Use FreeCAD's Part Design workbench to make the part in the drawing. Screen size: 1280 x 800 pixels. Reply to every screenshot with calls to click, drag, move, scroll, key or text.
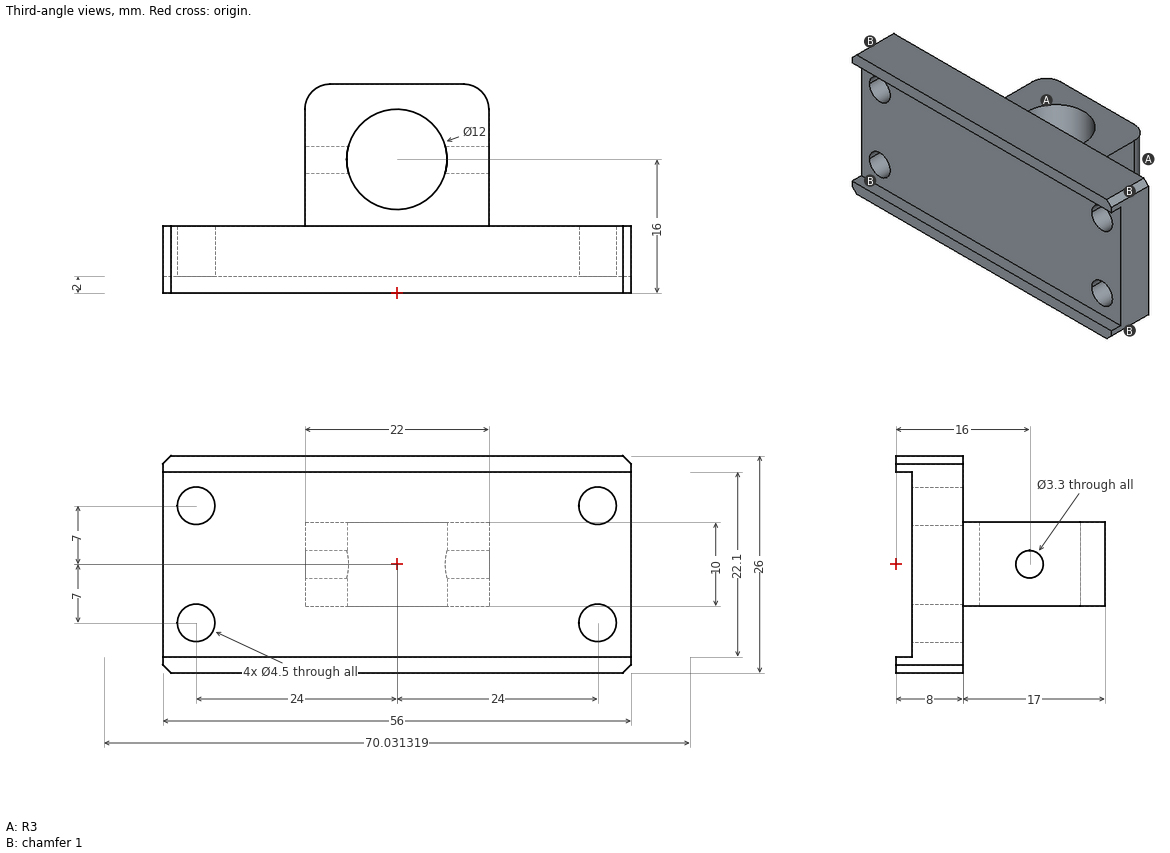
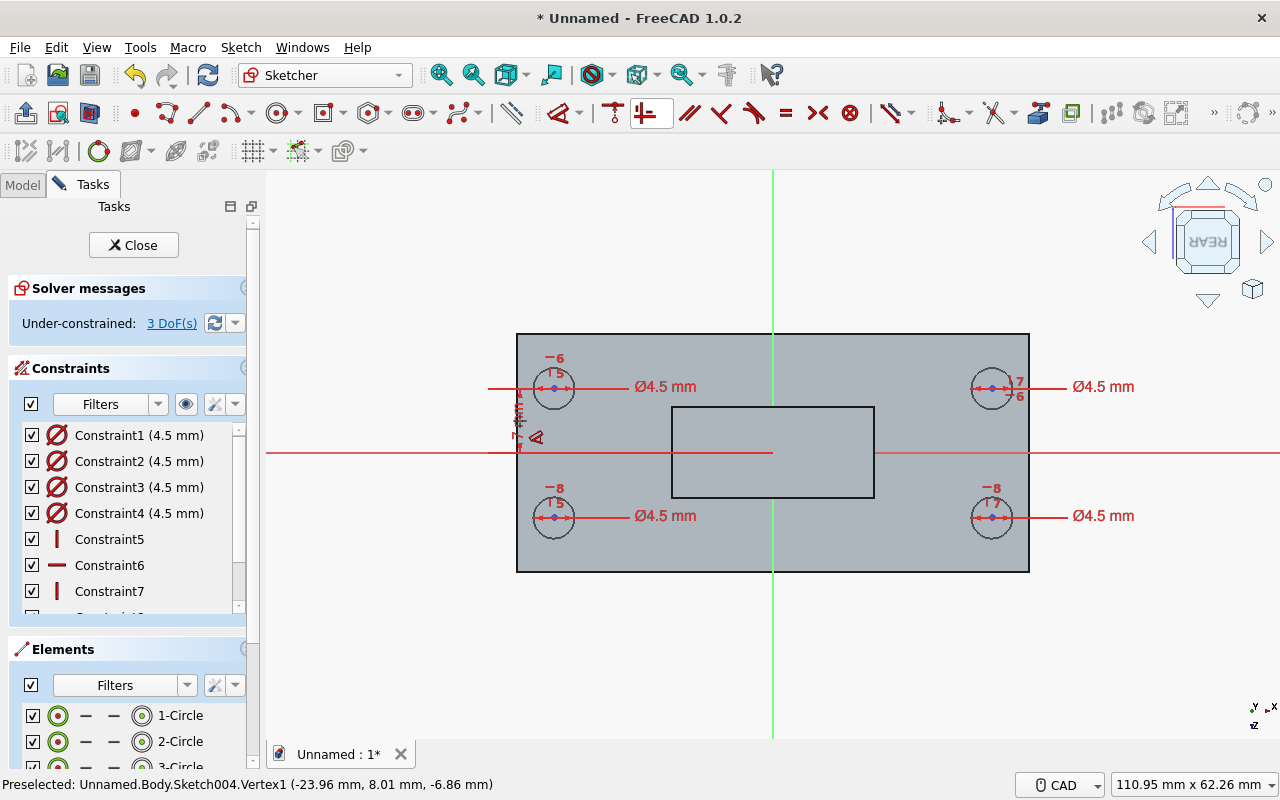
click(554, 518)
click(520, 485)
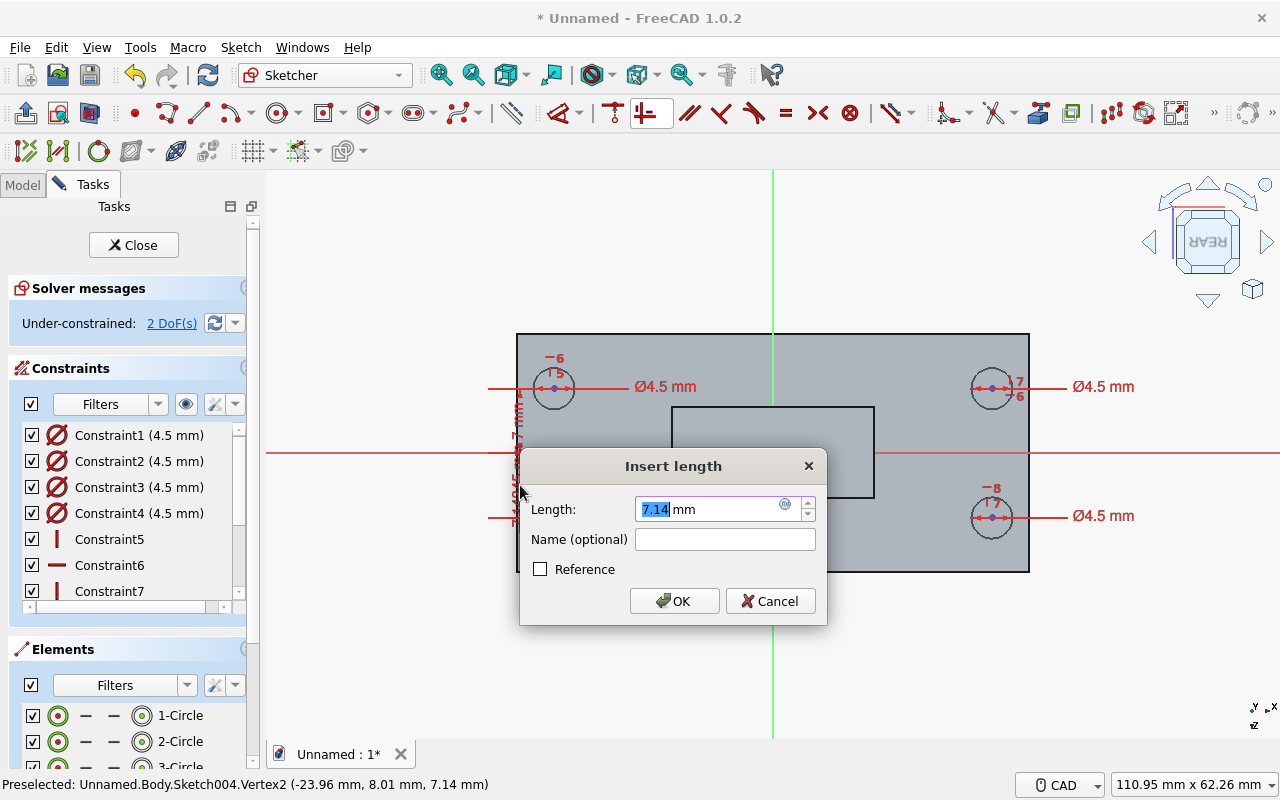
text(7)
key(Return)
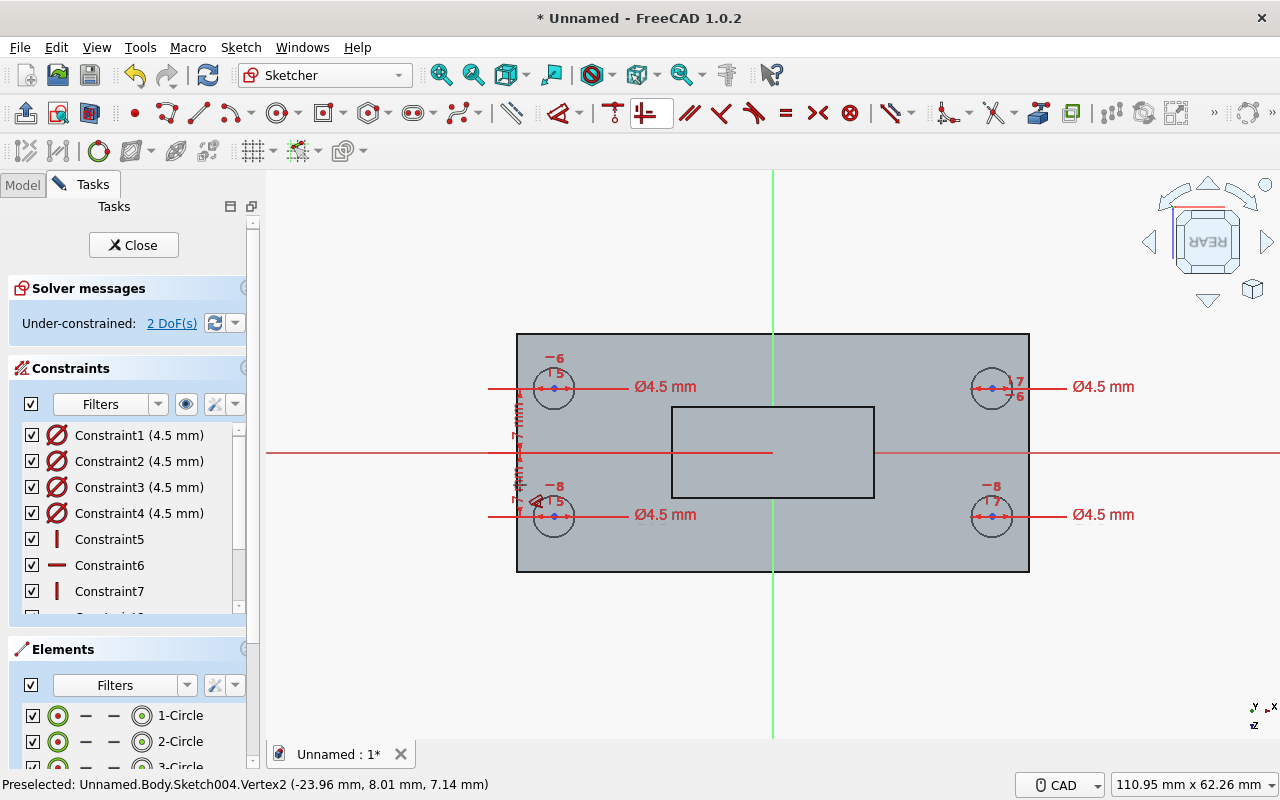
click(554, 389)
click(663, 355)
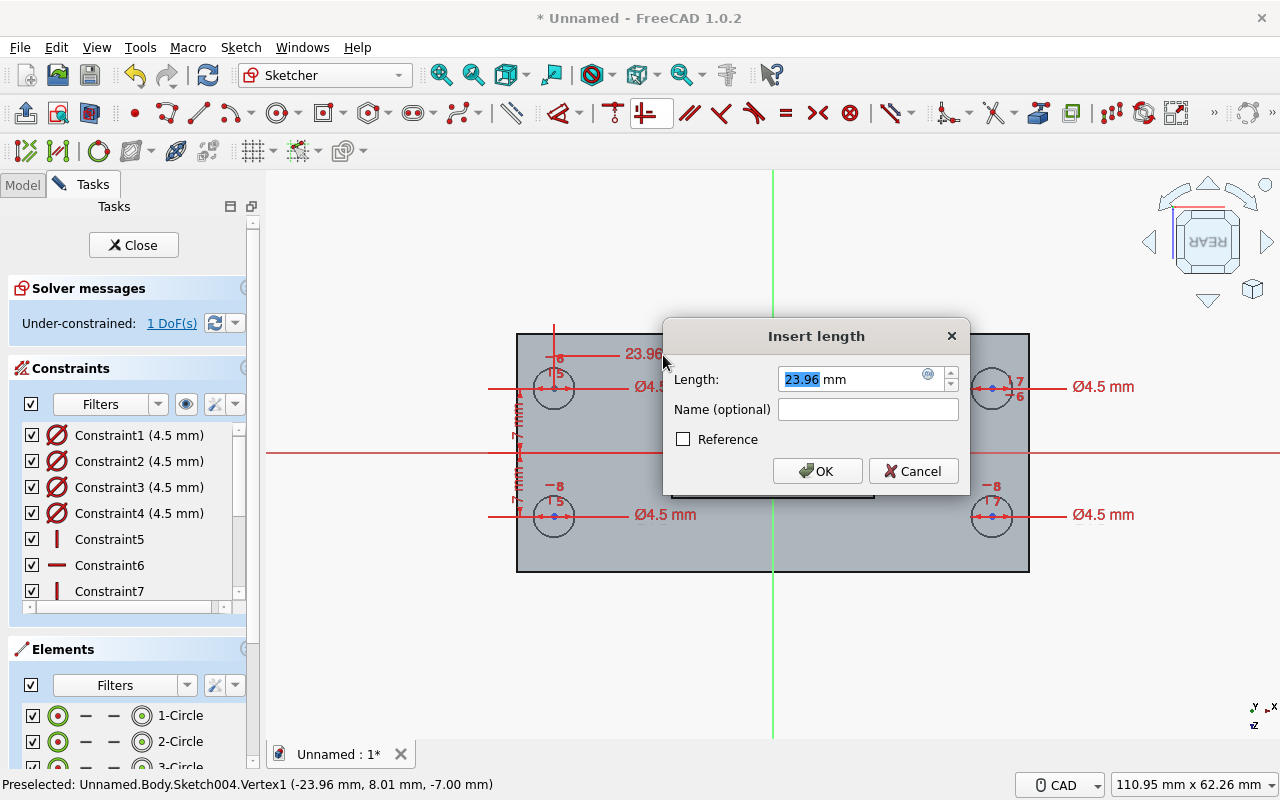
text(24)
key(Return)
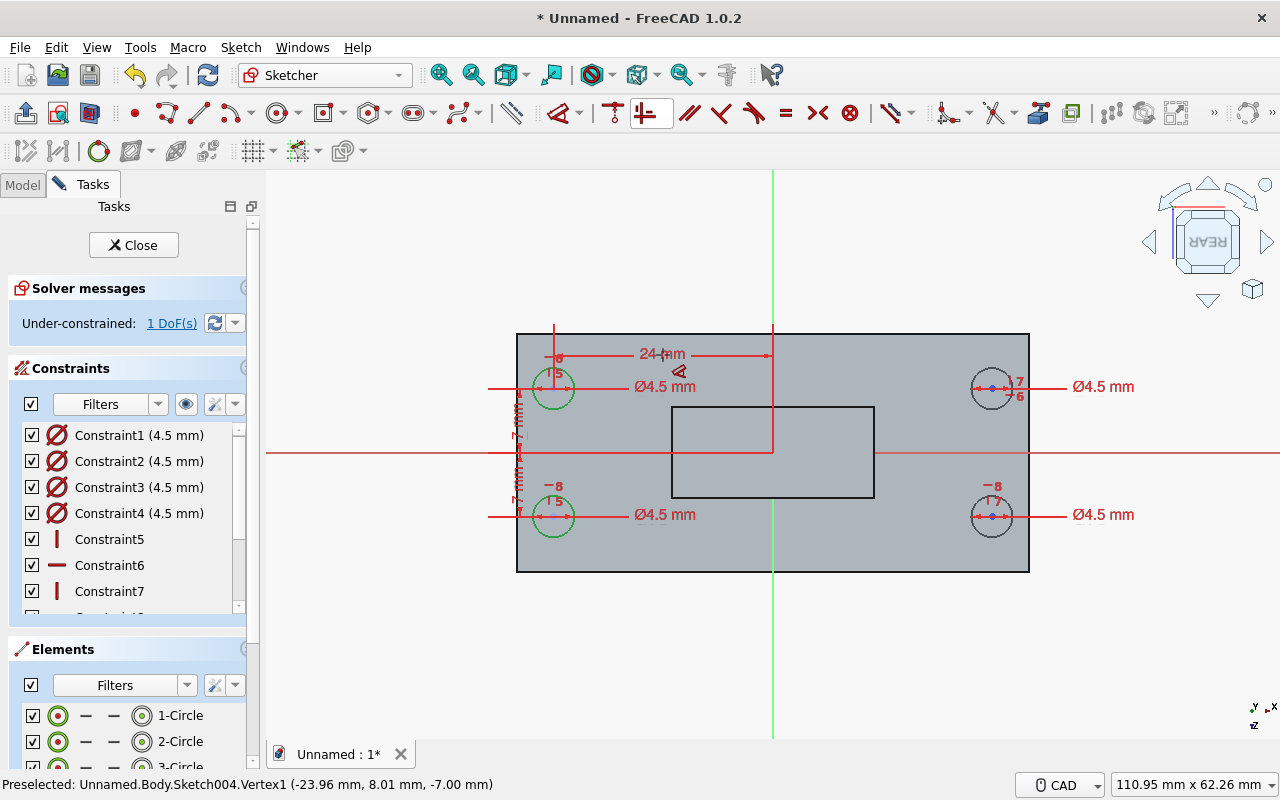
click(992, 389)
click(882, 355)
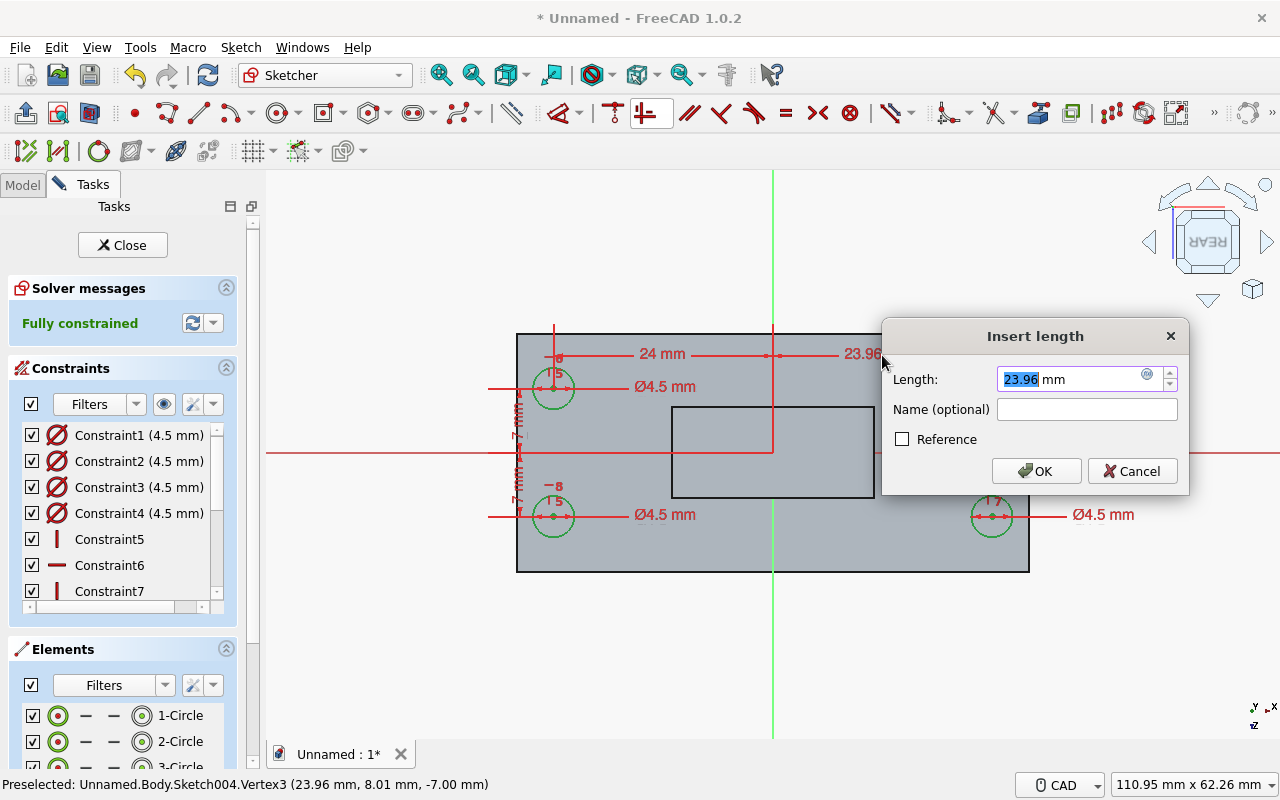
text(24)
key(Return)
key(Escape)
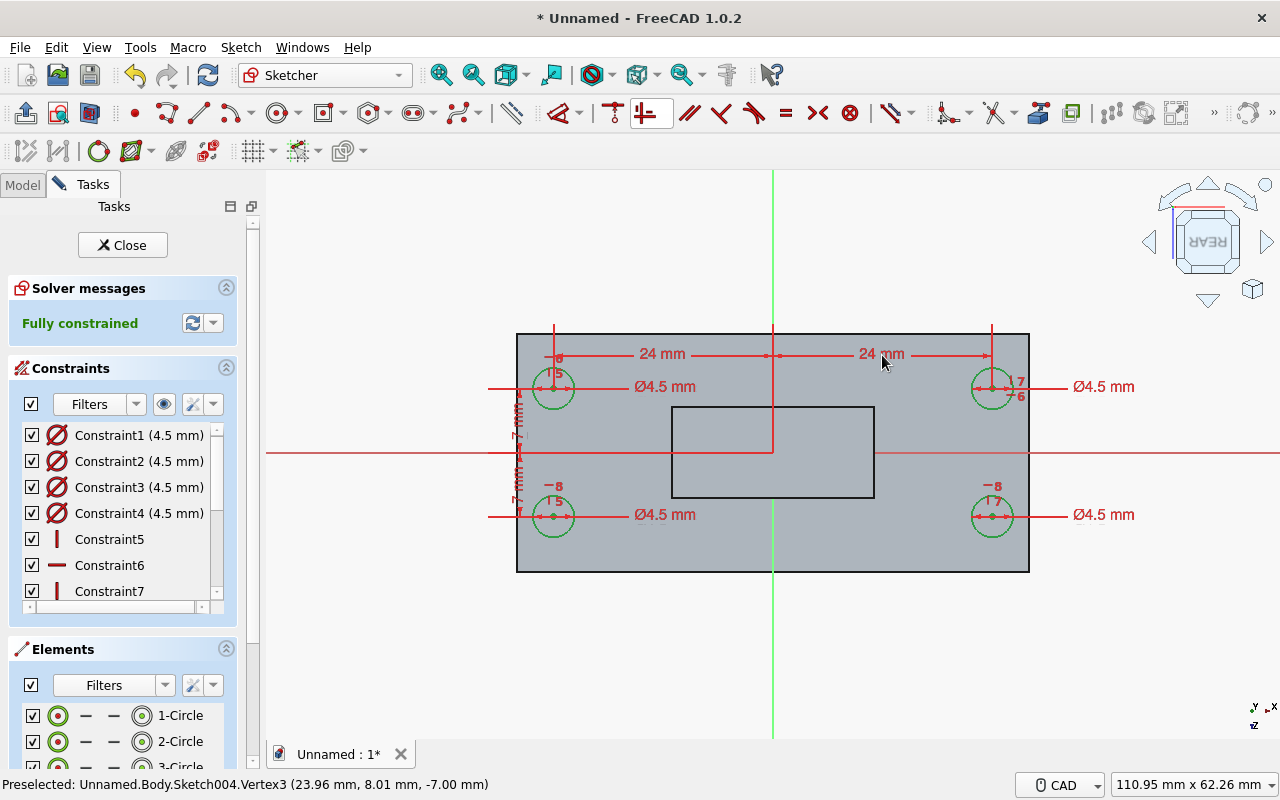
click(123, 245)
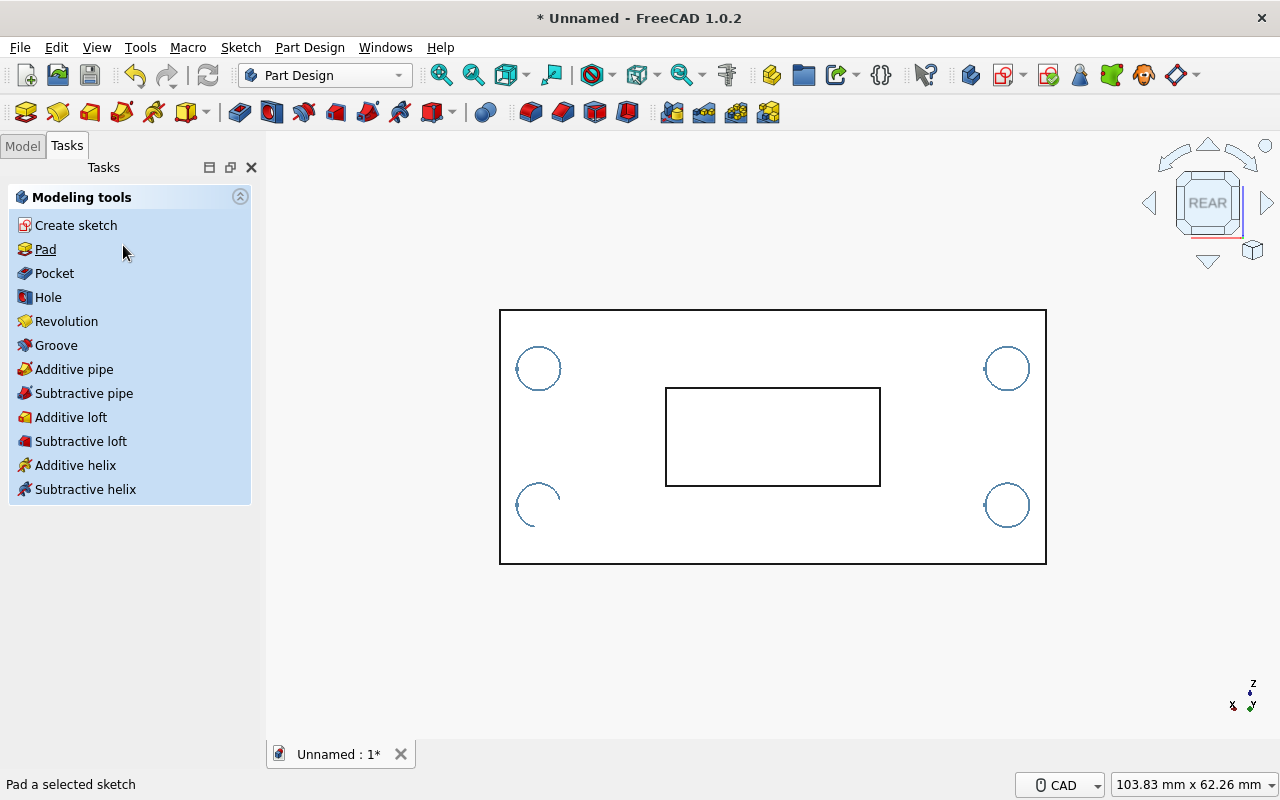
click(272, 112)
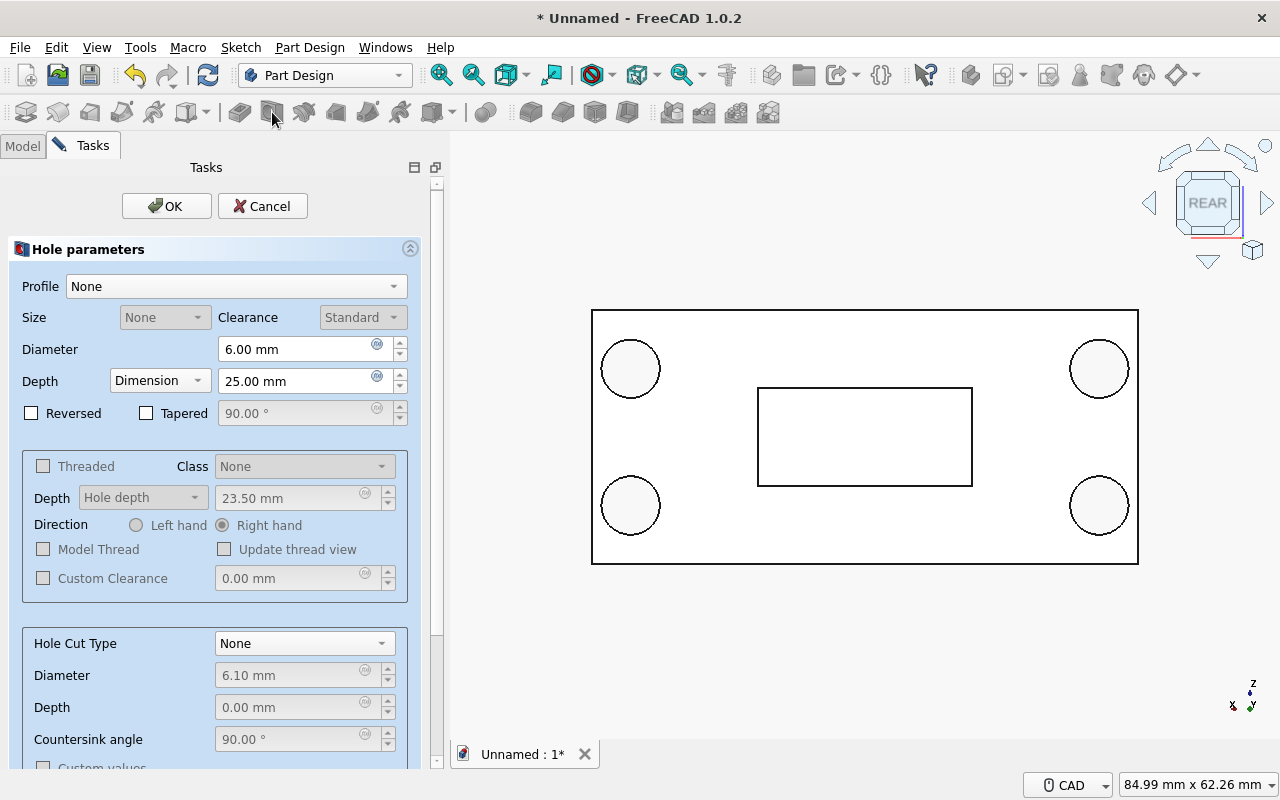
triple_click(305, 349)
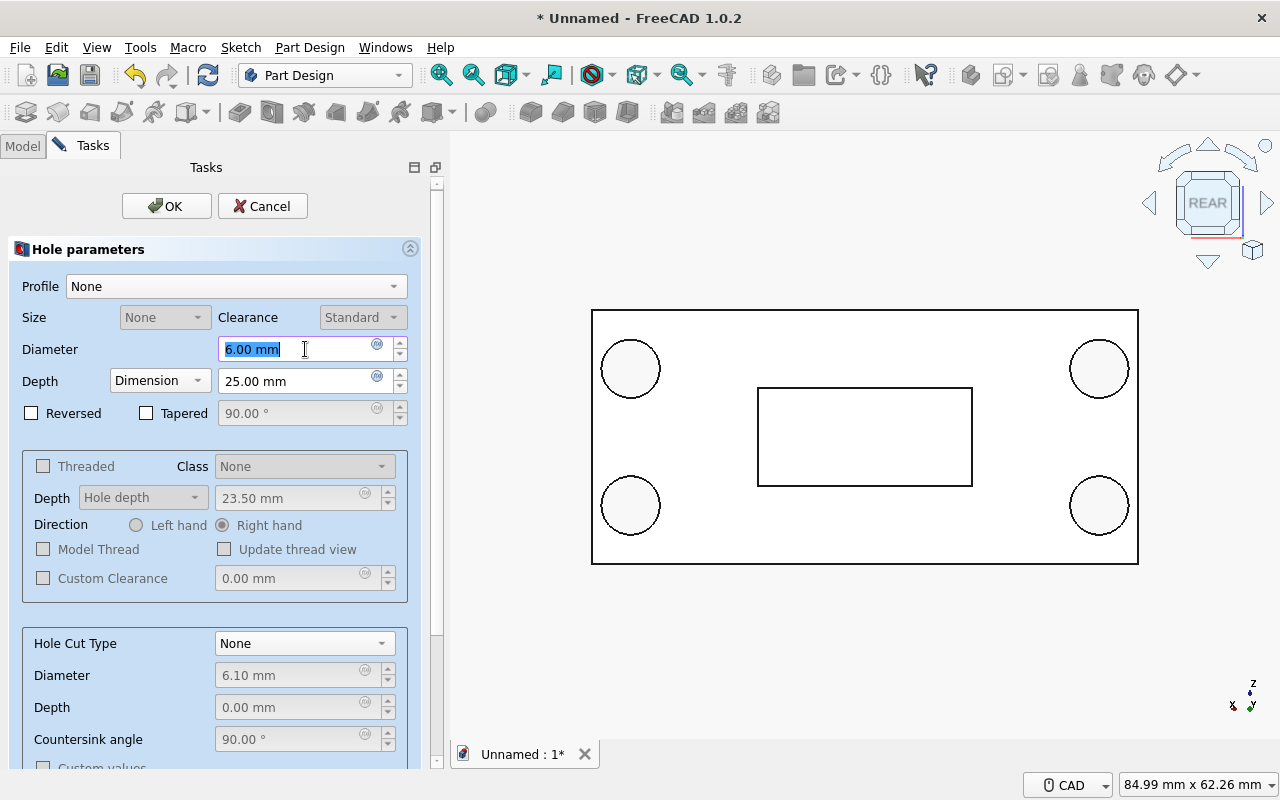
text(4.5)
key(Tab)